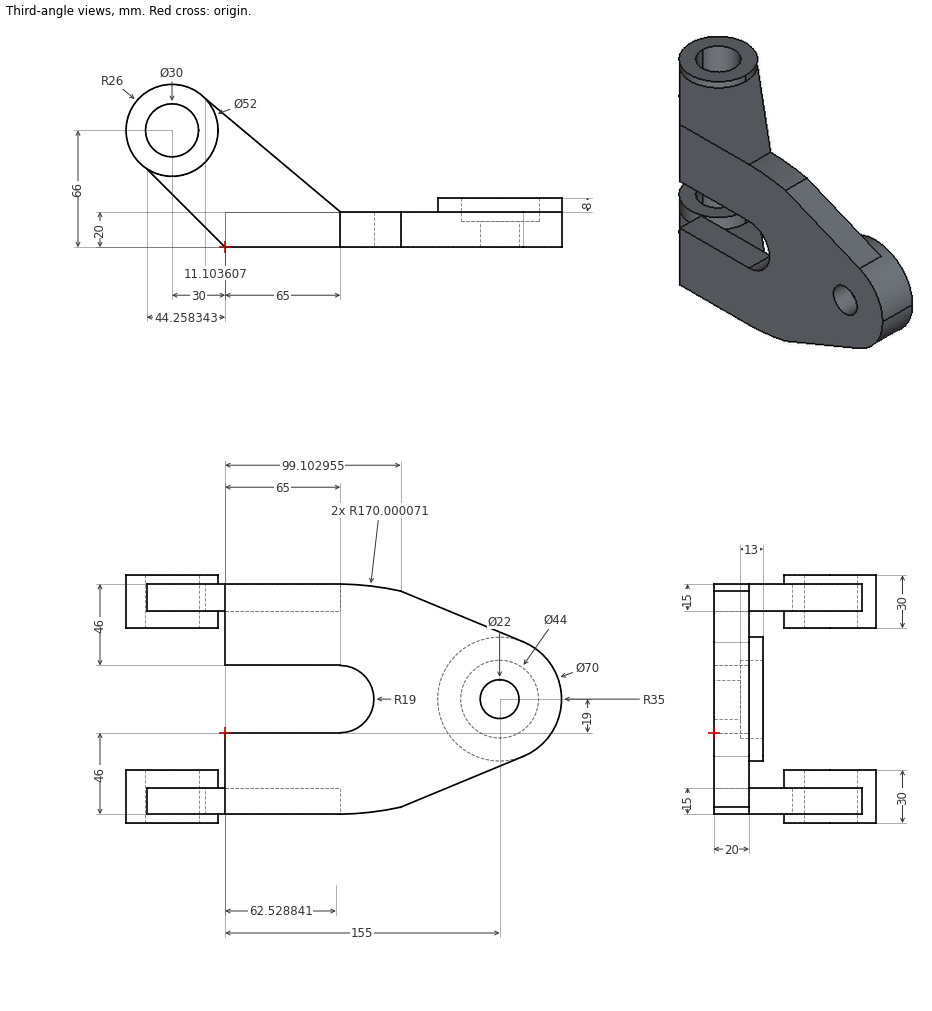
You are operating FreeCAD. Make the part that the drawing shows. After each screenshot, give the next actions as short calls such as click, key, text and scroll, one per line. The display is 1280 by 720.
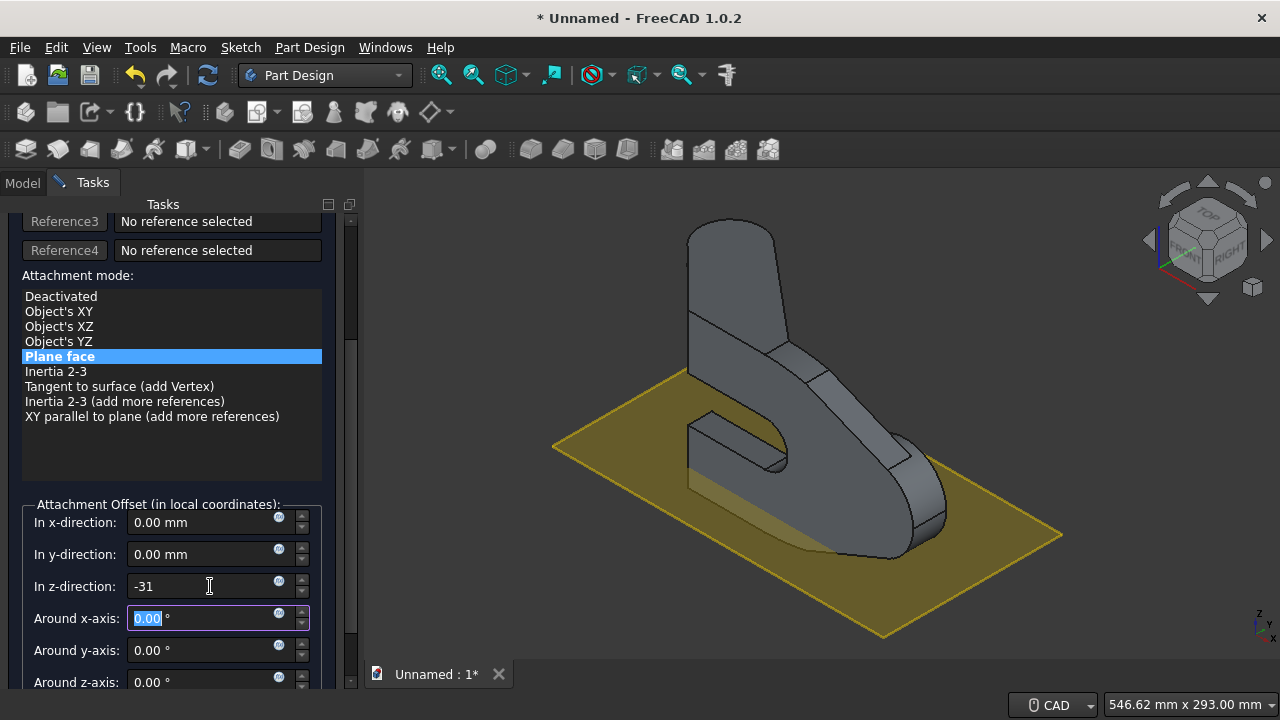
scroll(351, 451, up, 4)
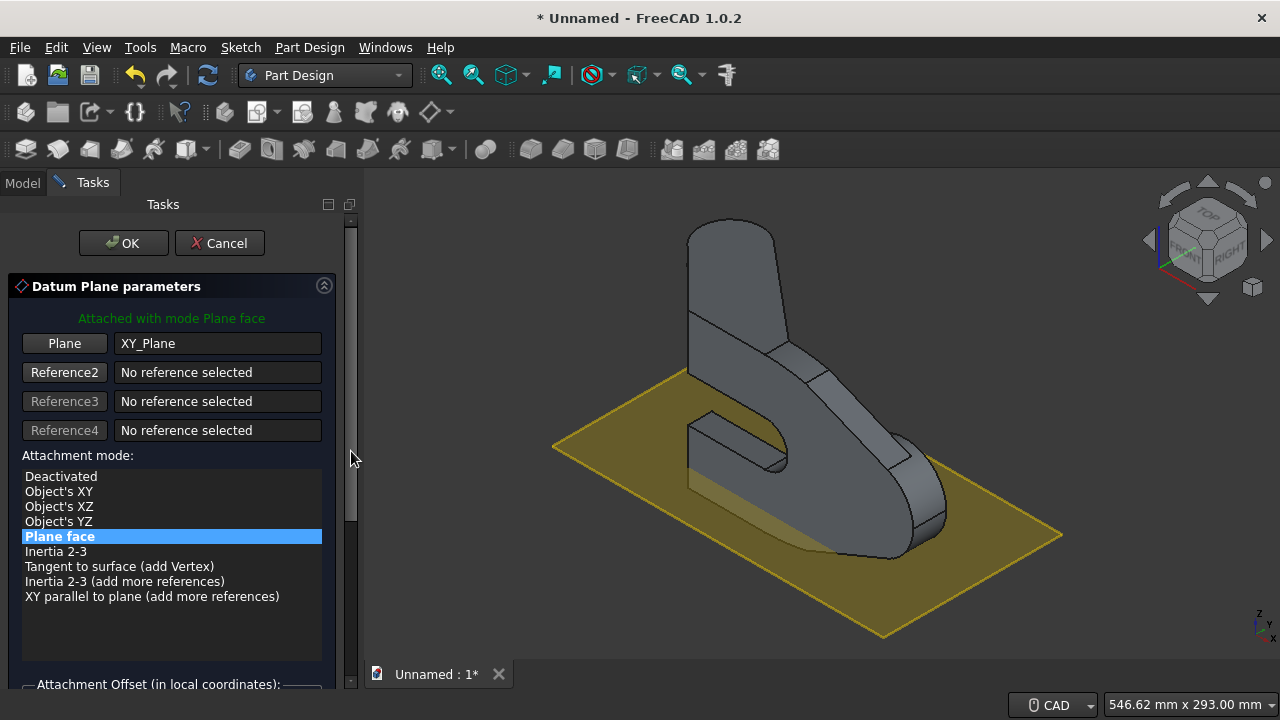
click(124, 243)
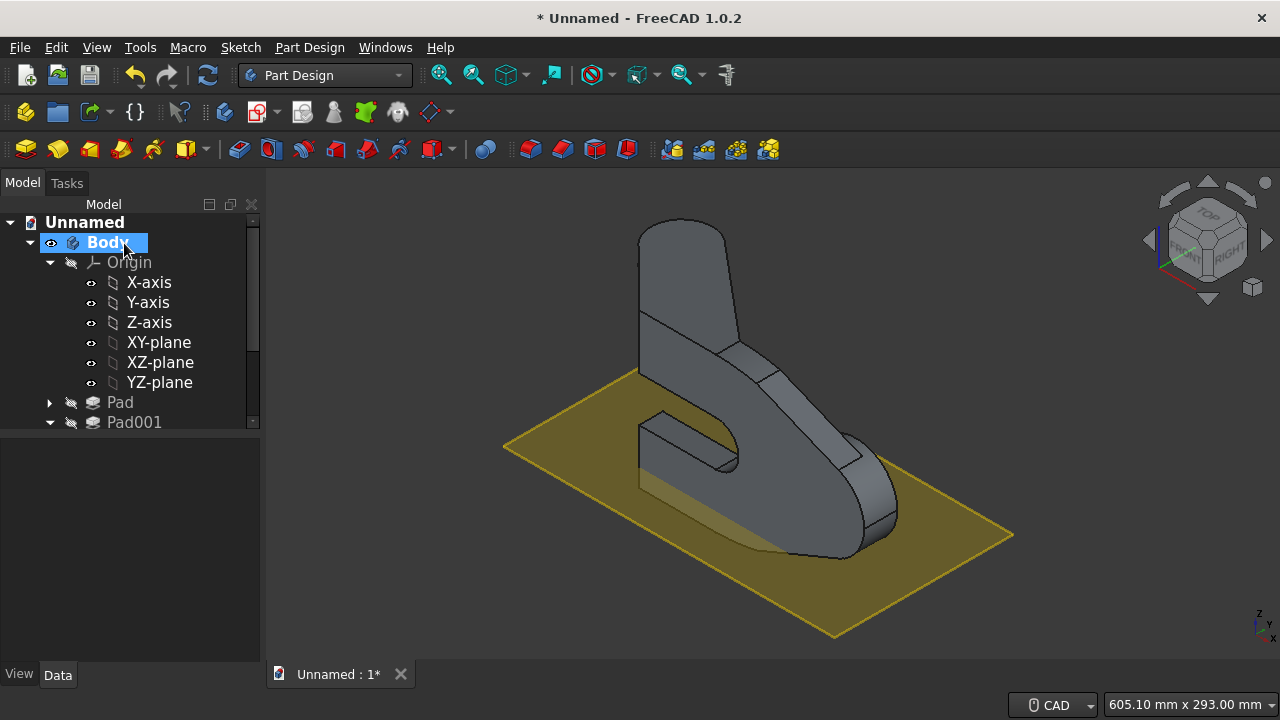
scroll(100, 318, down, 3)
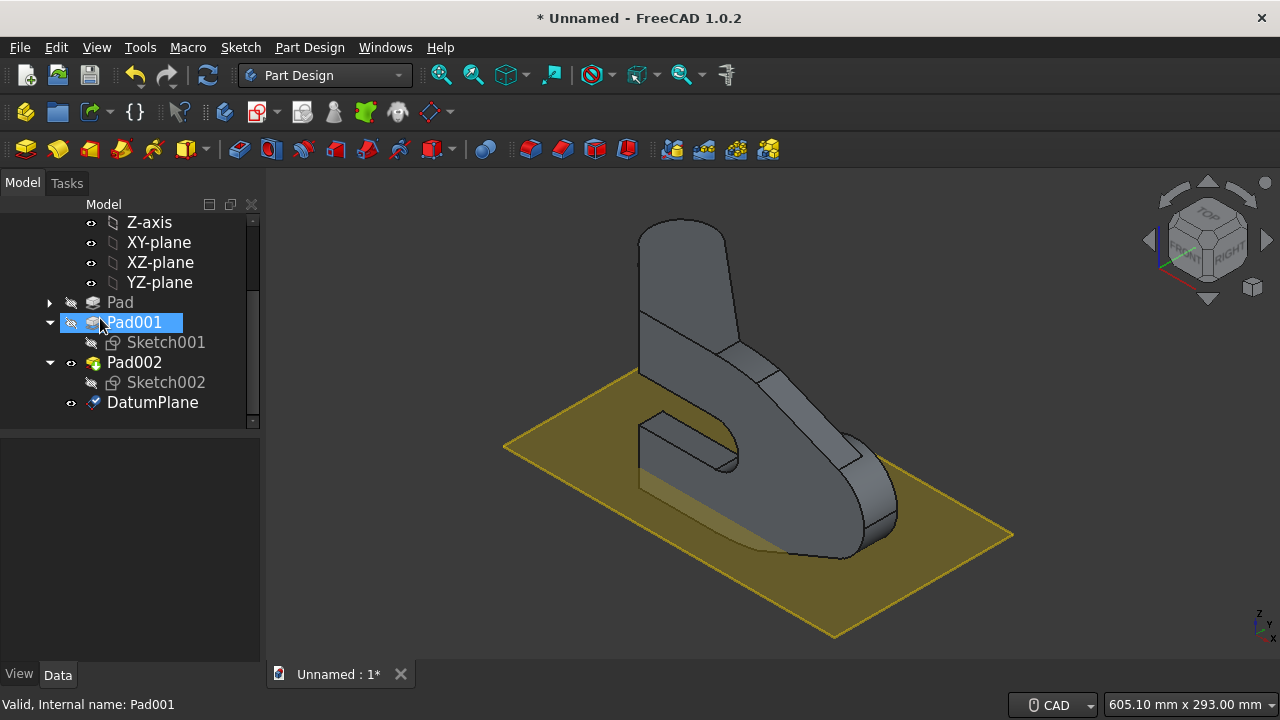
click(116, 403)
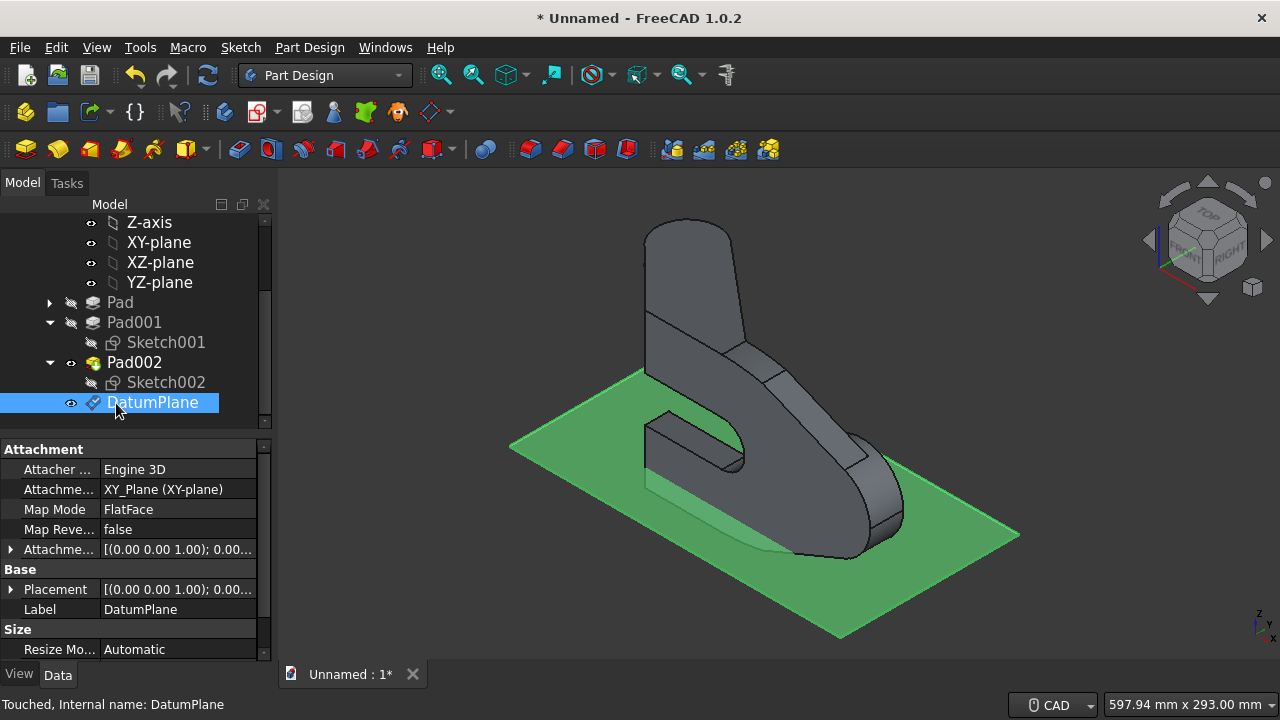
click(258, 112)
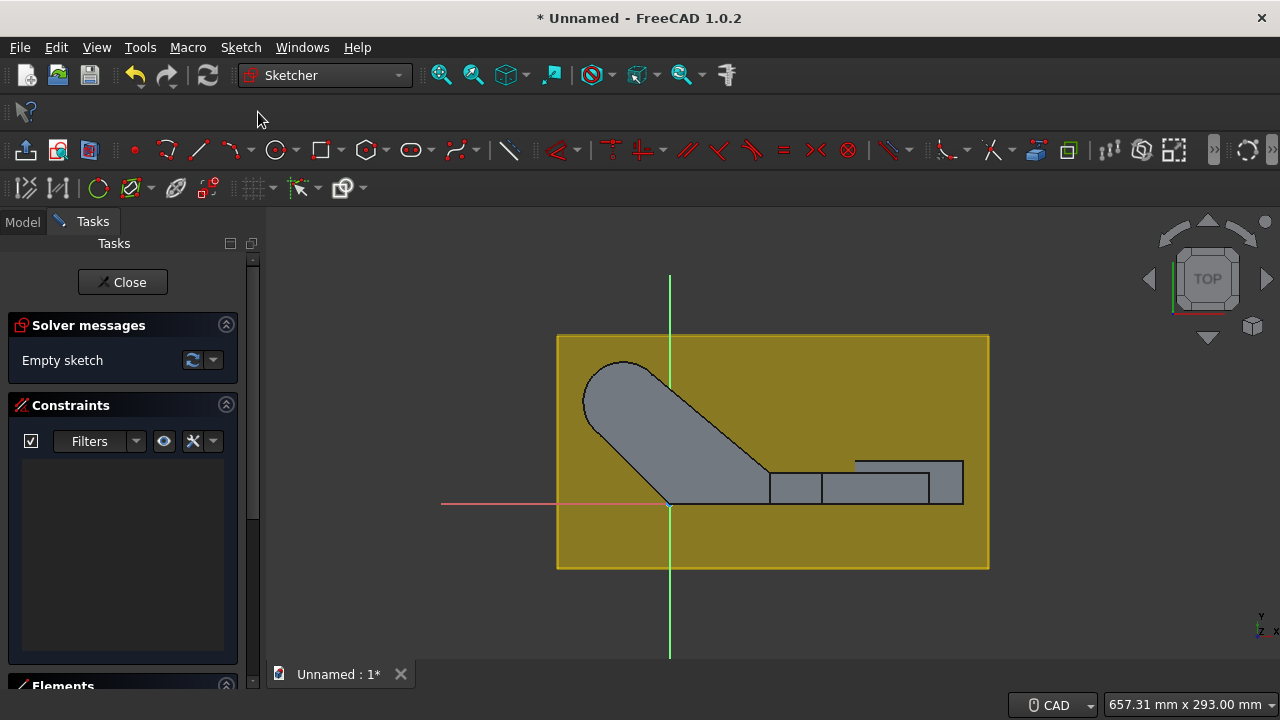
key(q)
key(s)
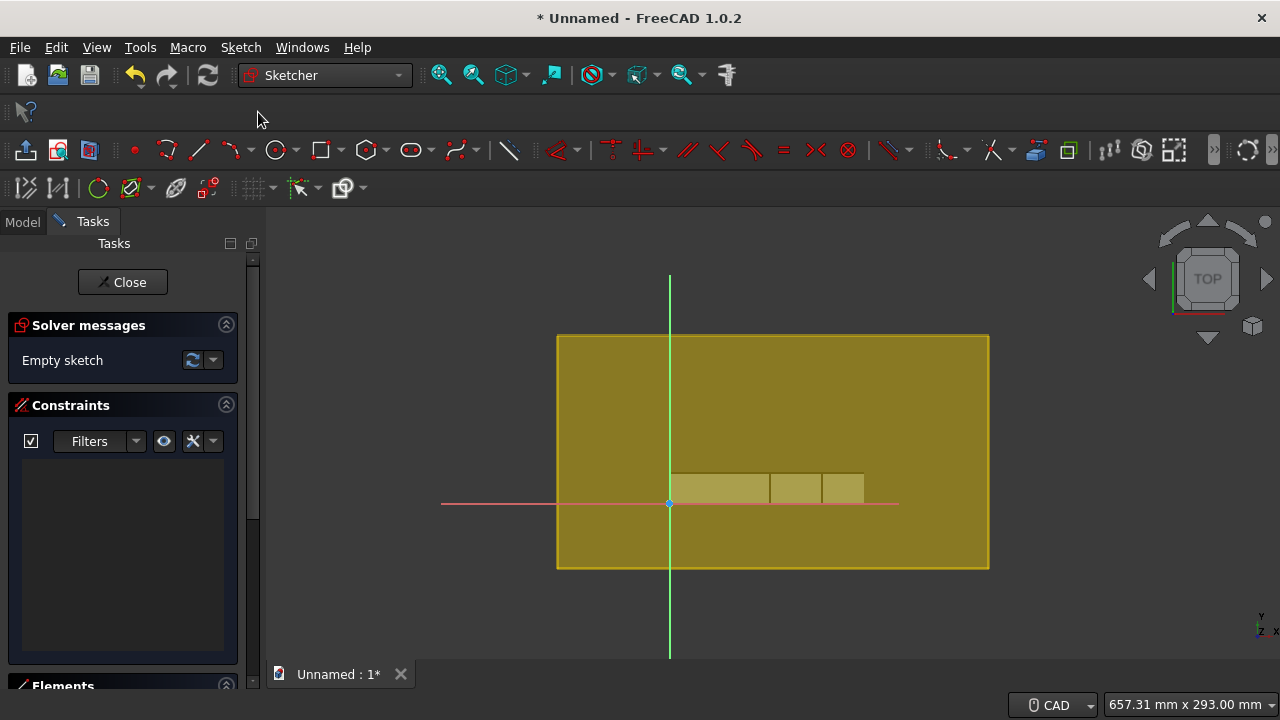
scroll(662, 444, up, 4)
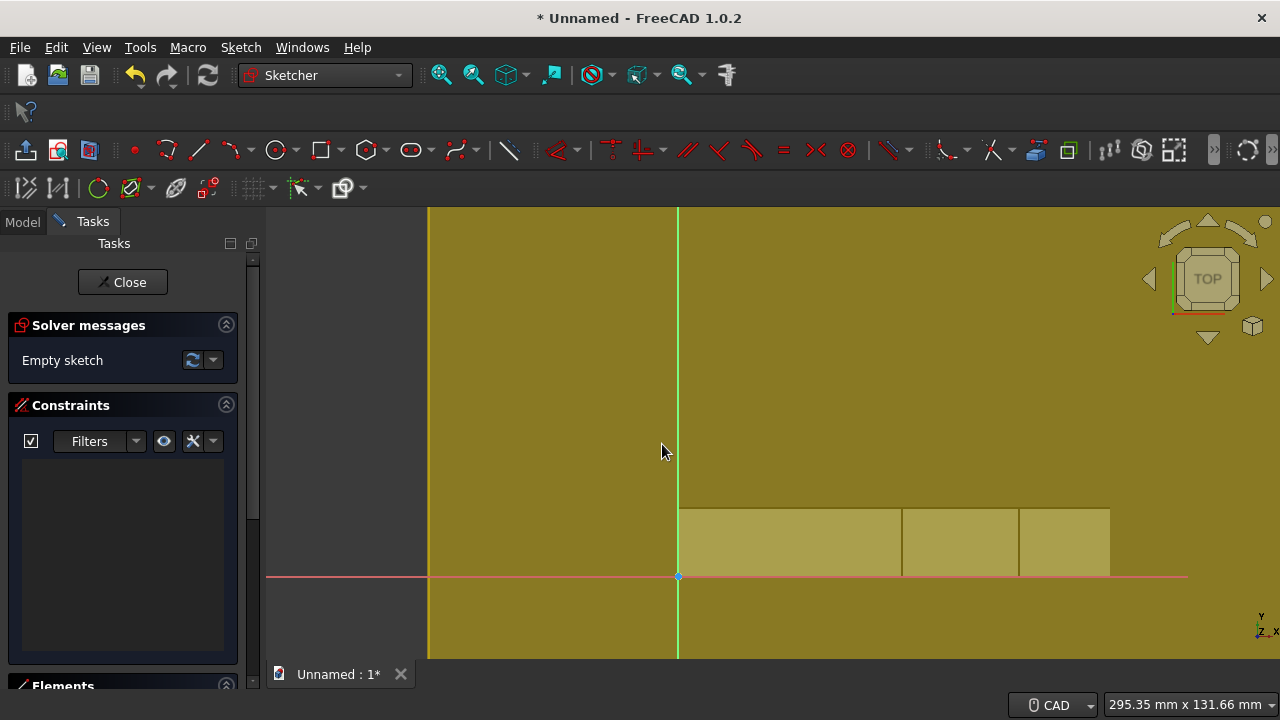
click(168, 150)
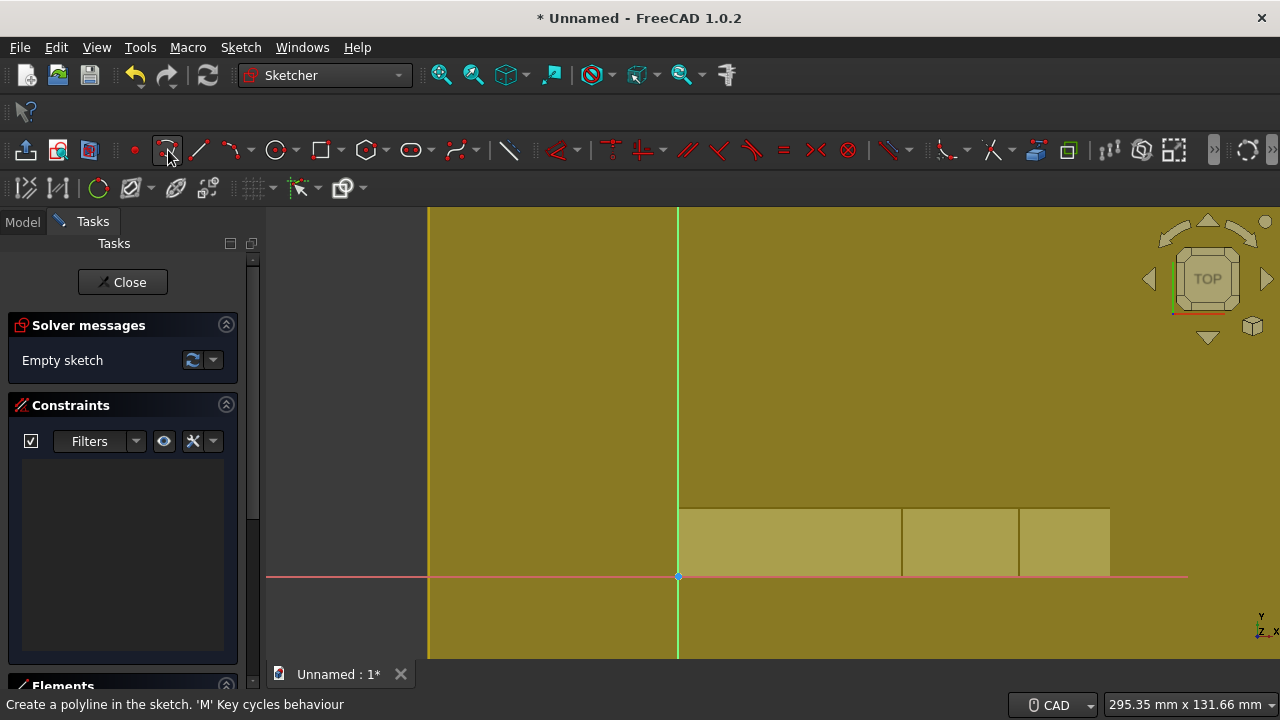
click(640, 289)
click(902, 508)
click(902, 577)
click(678, 577)
click(526, 425)
right_click(526, 425)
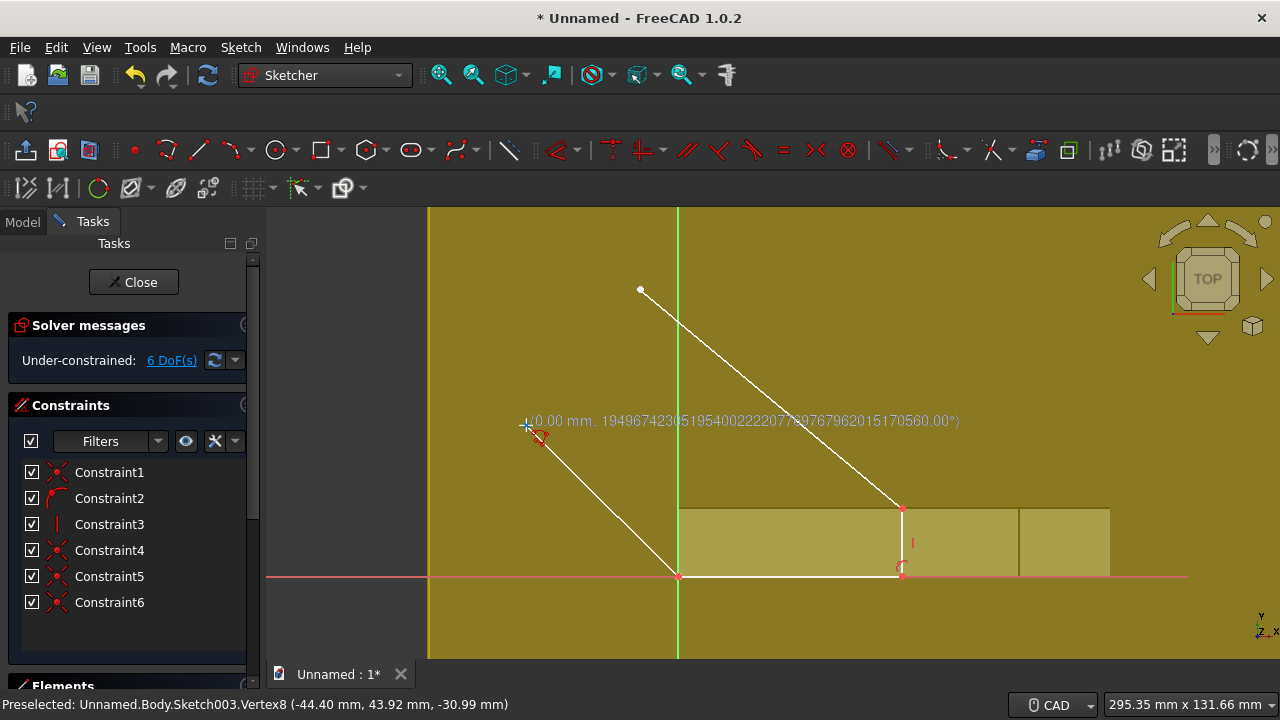
click(232, 150)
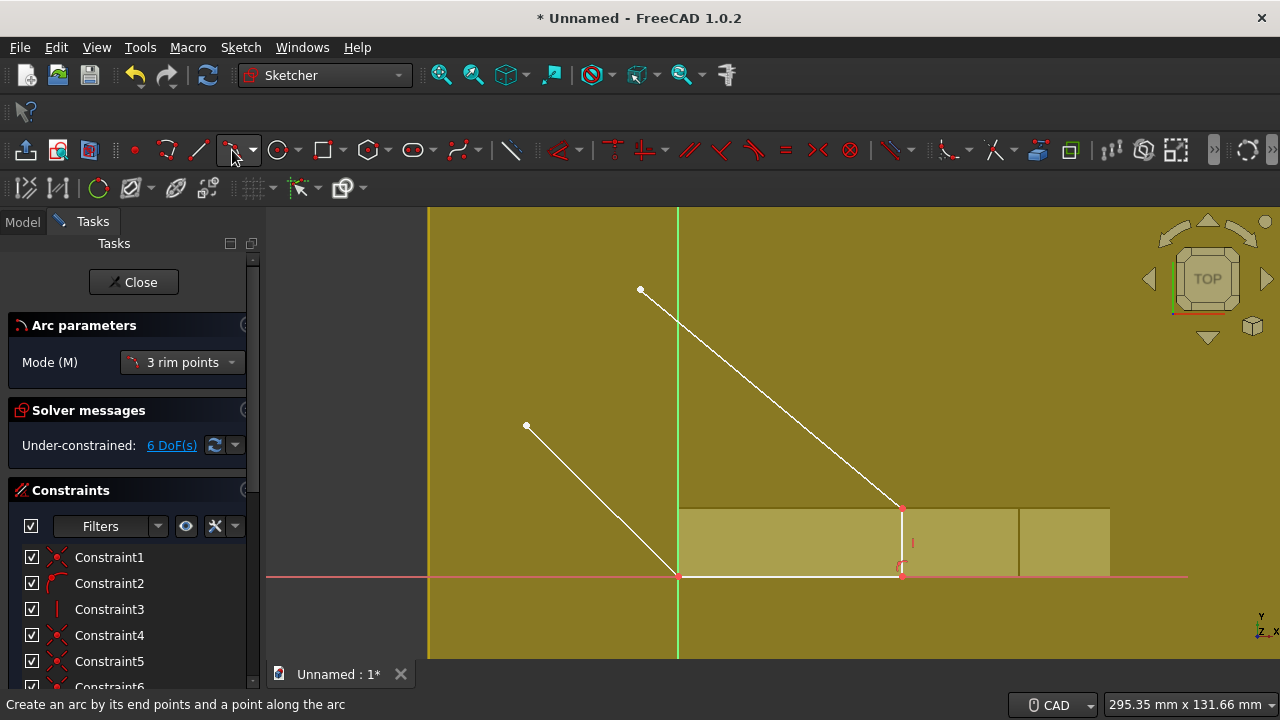
click(526, 426)
click(640, 290)
click(507, 293)
key(Escape)